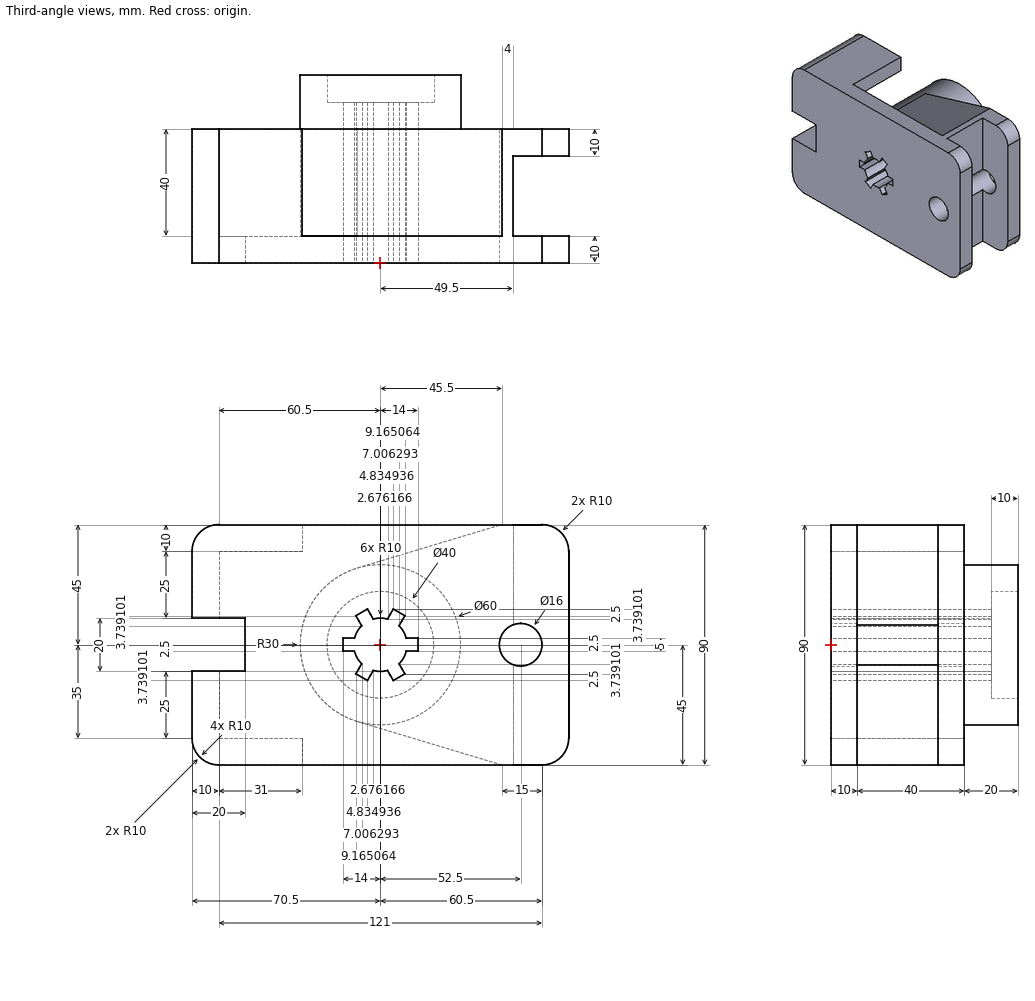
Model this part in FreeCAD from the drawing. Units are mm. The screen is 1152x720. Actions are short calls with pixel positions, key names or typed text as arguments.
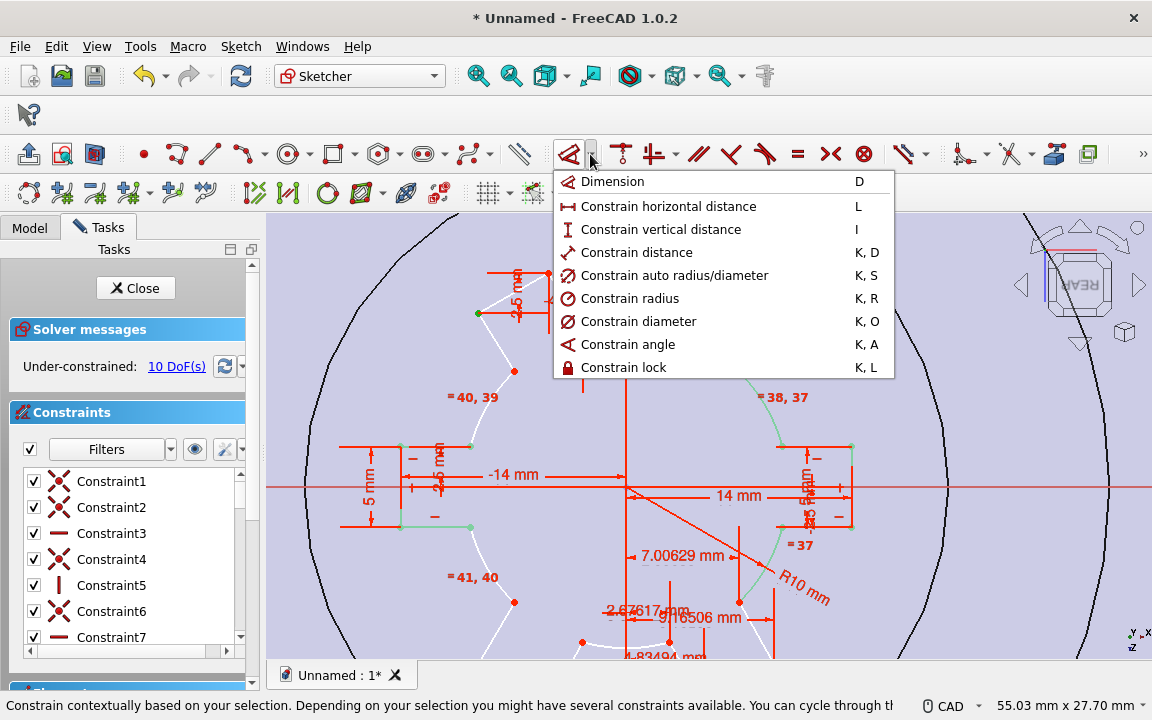
click(724, 206)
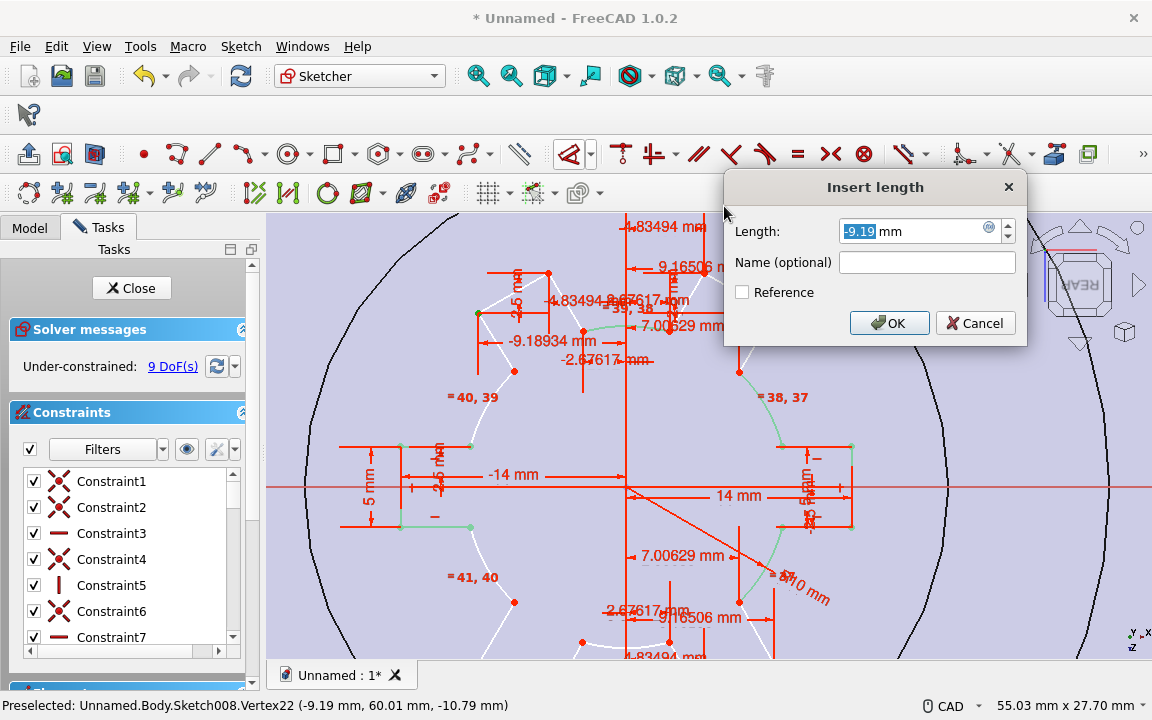
text(-9.165064)
key(Return)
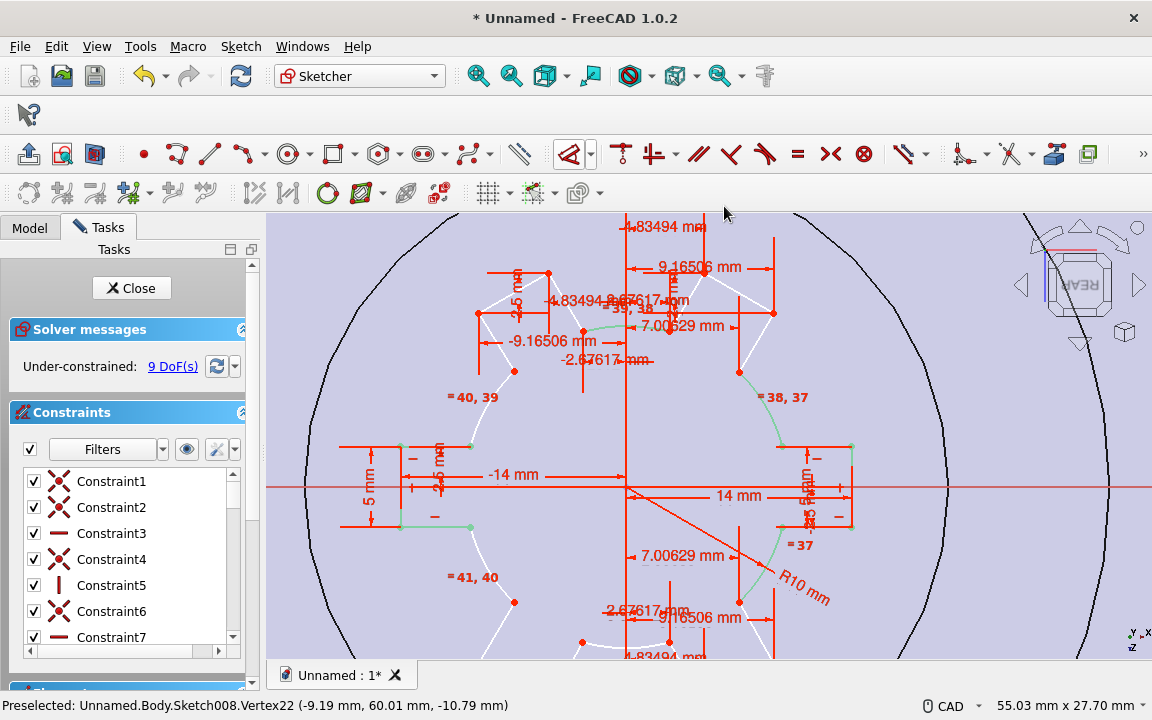
click(515, 371)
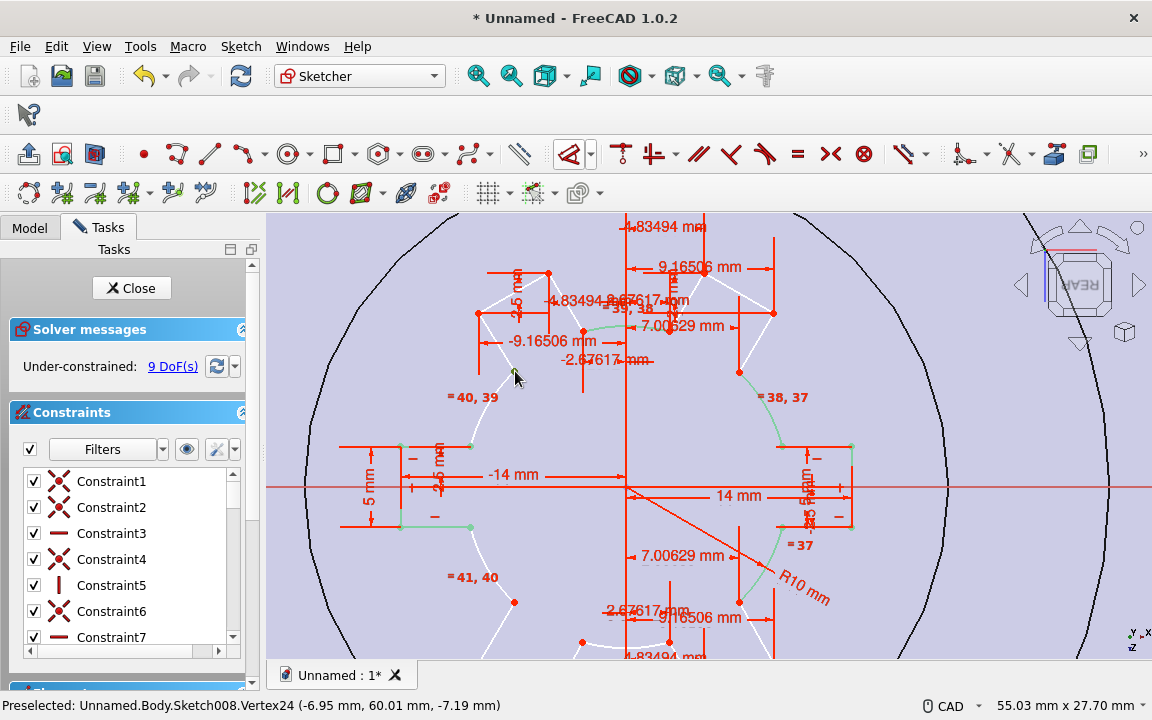
click(590, 154)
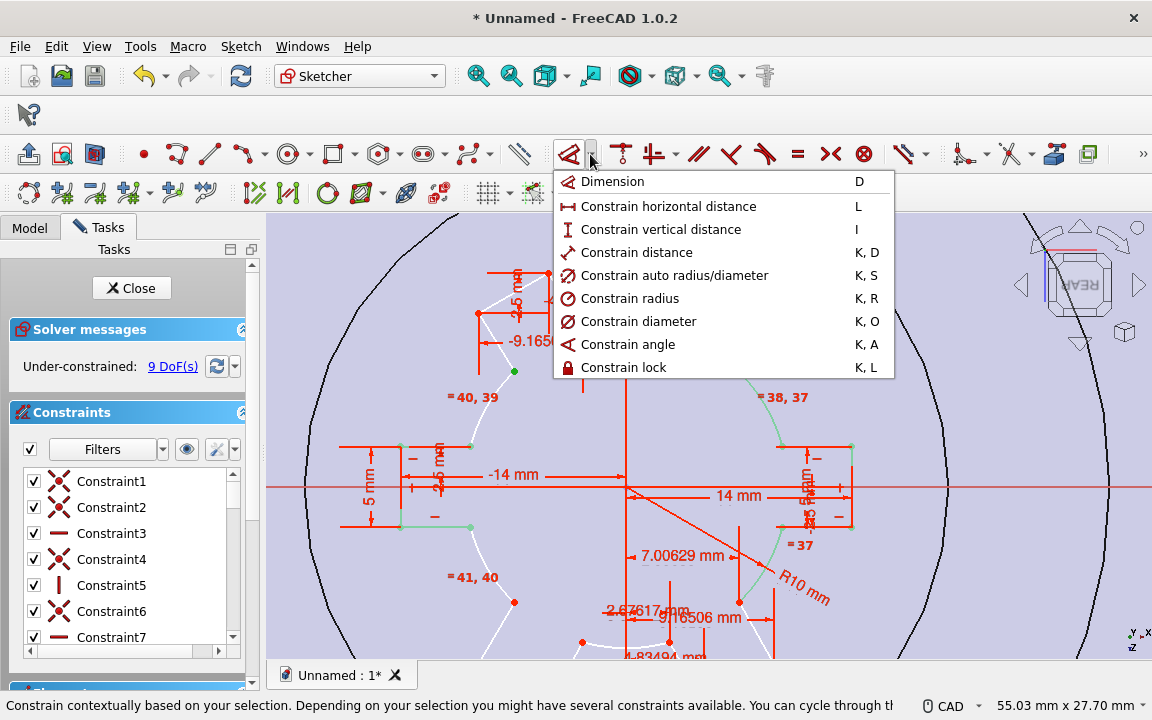
click(724, 206)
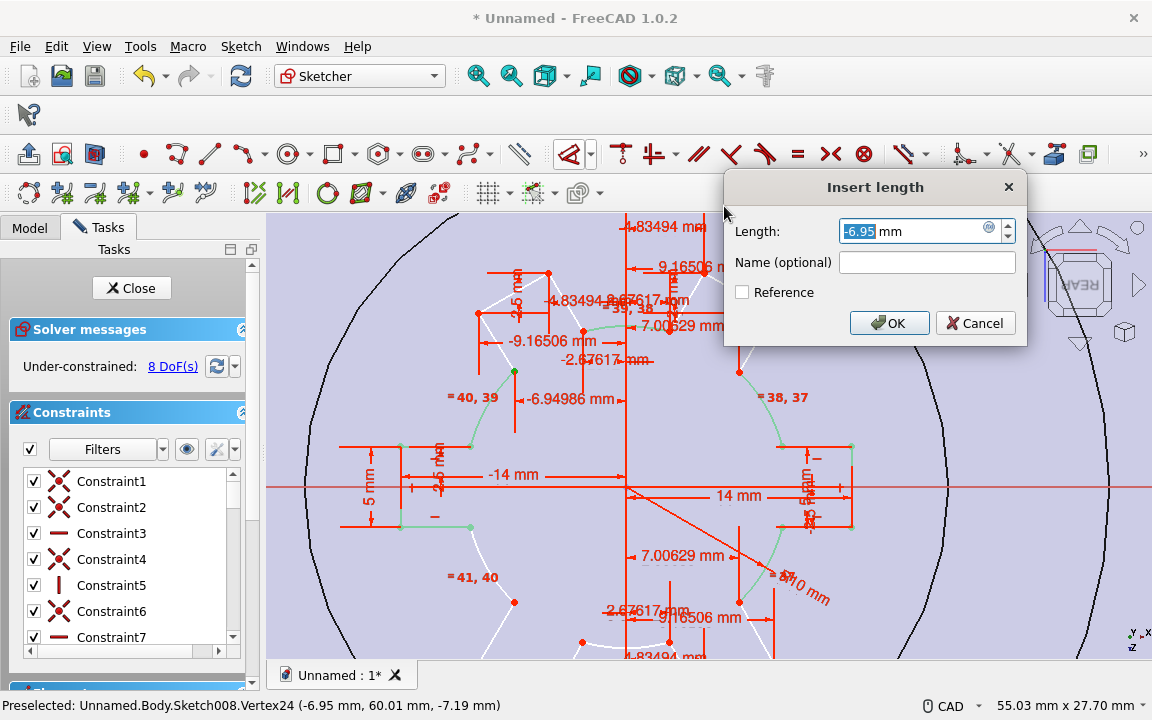
text(-7.006293)
key(Return)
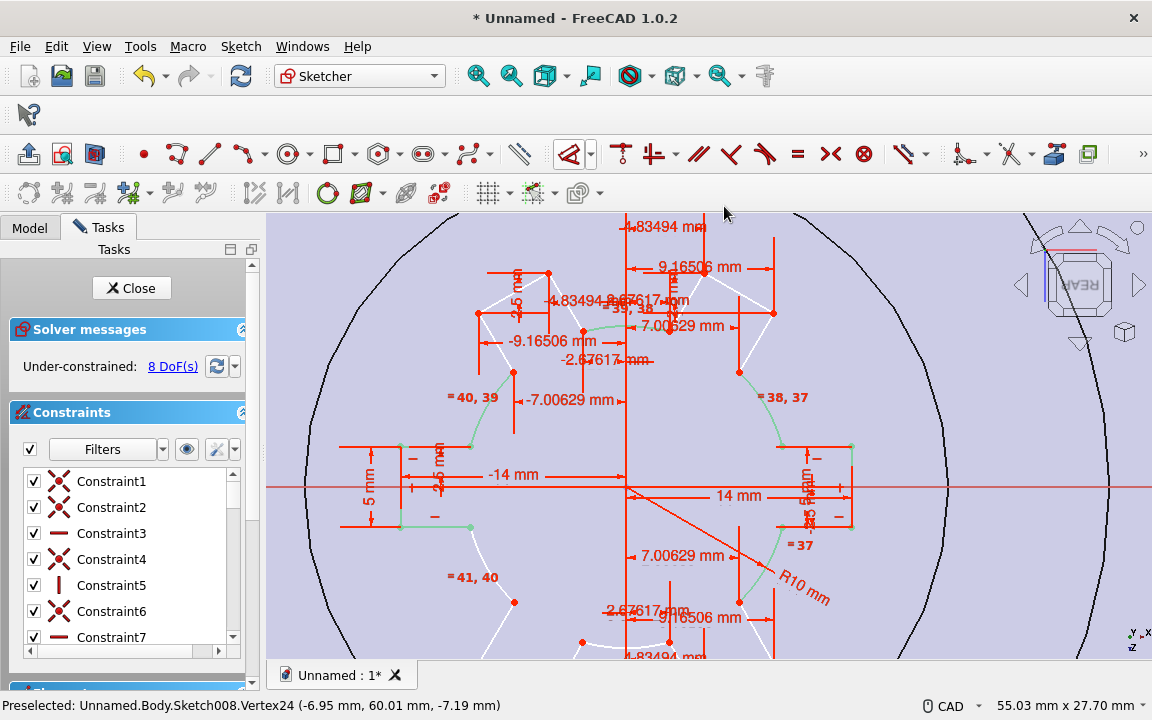
click(514, 603)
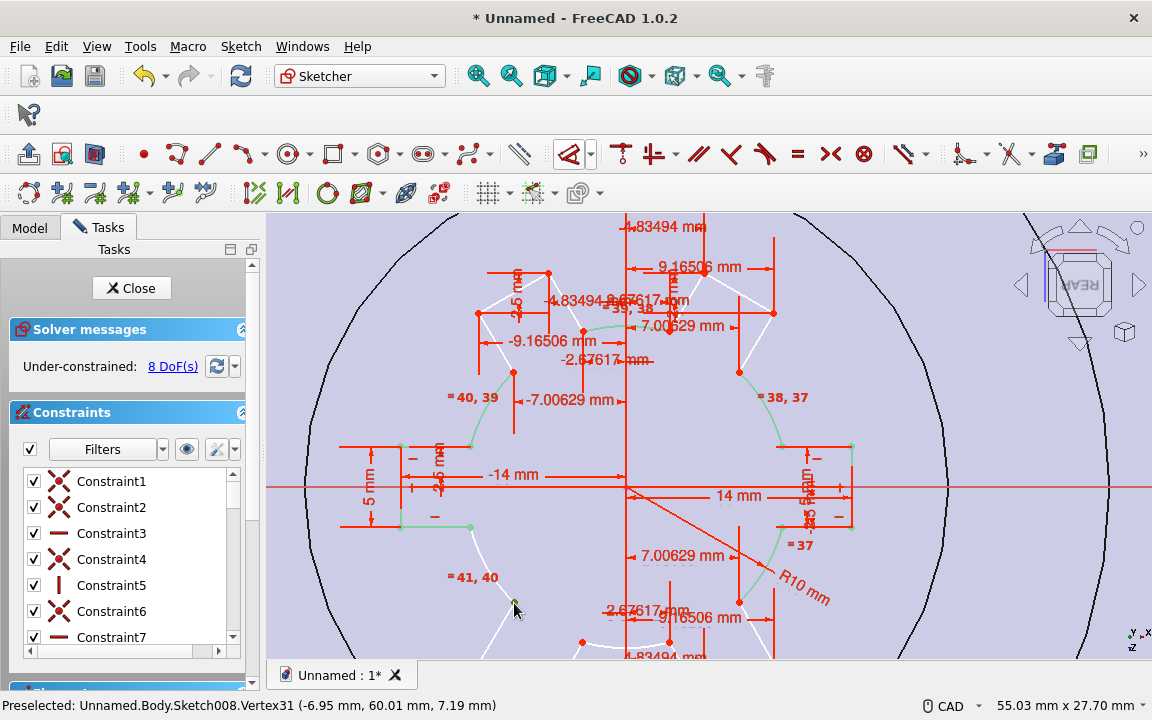
click(590, 154)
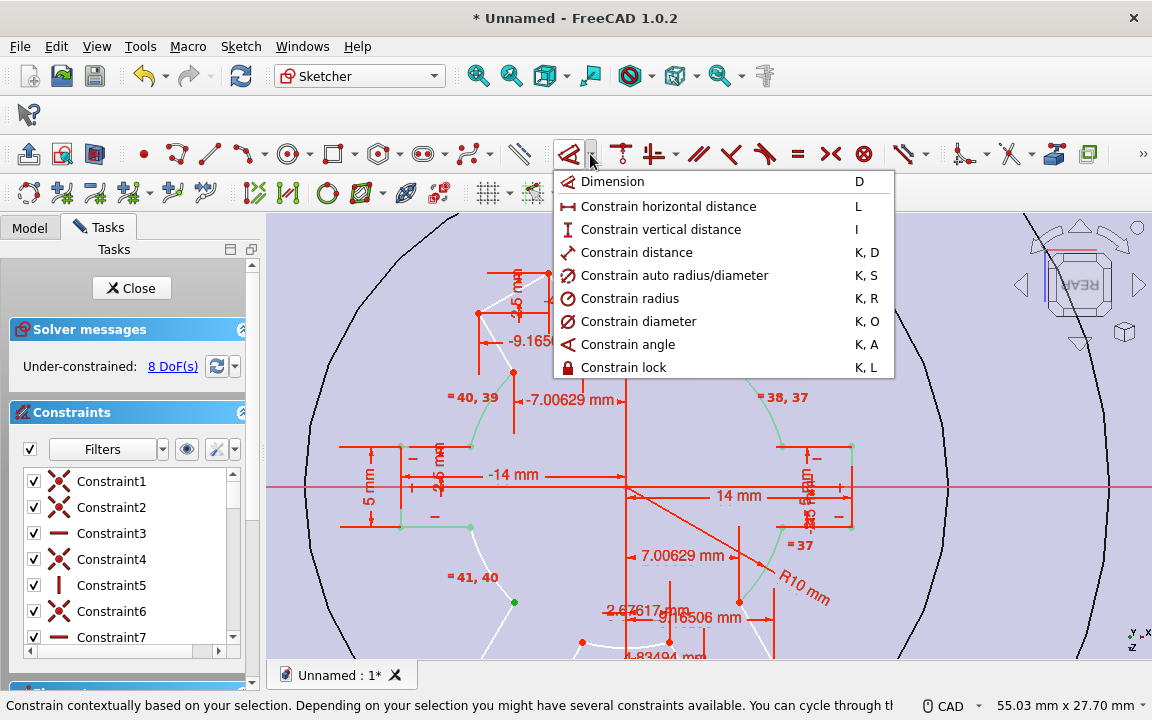
click(724, 206)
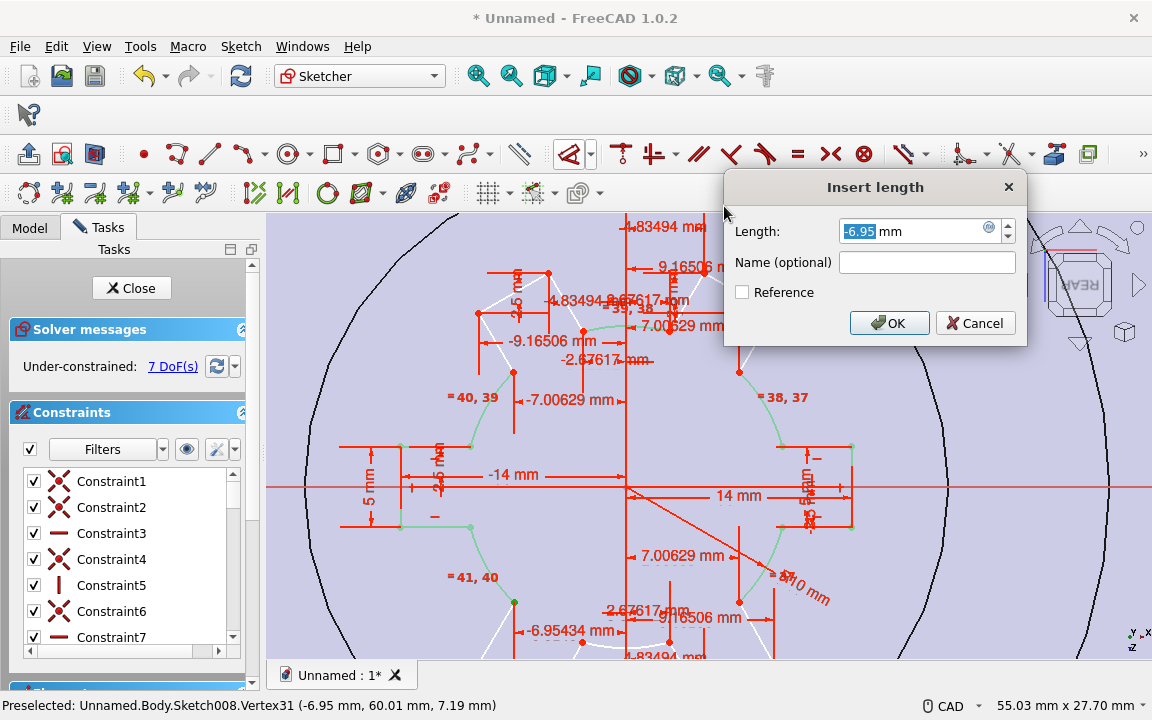
text(-7.006293)
key(Return)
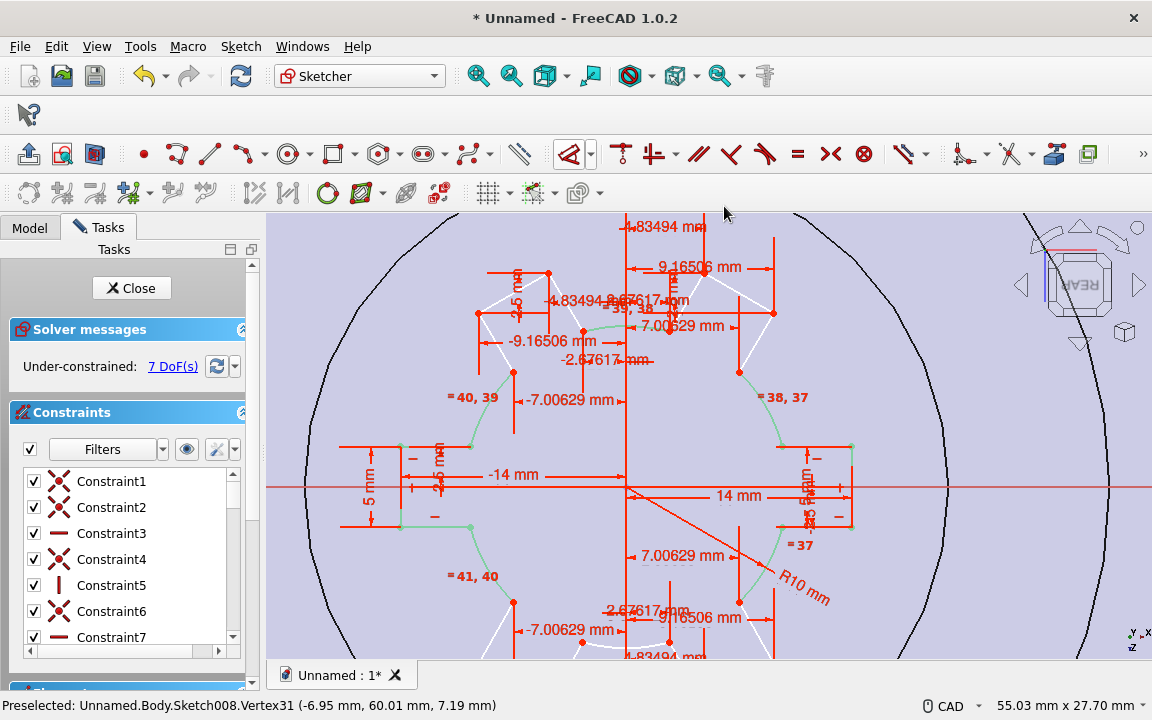
scroll(669, 332, down, 2)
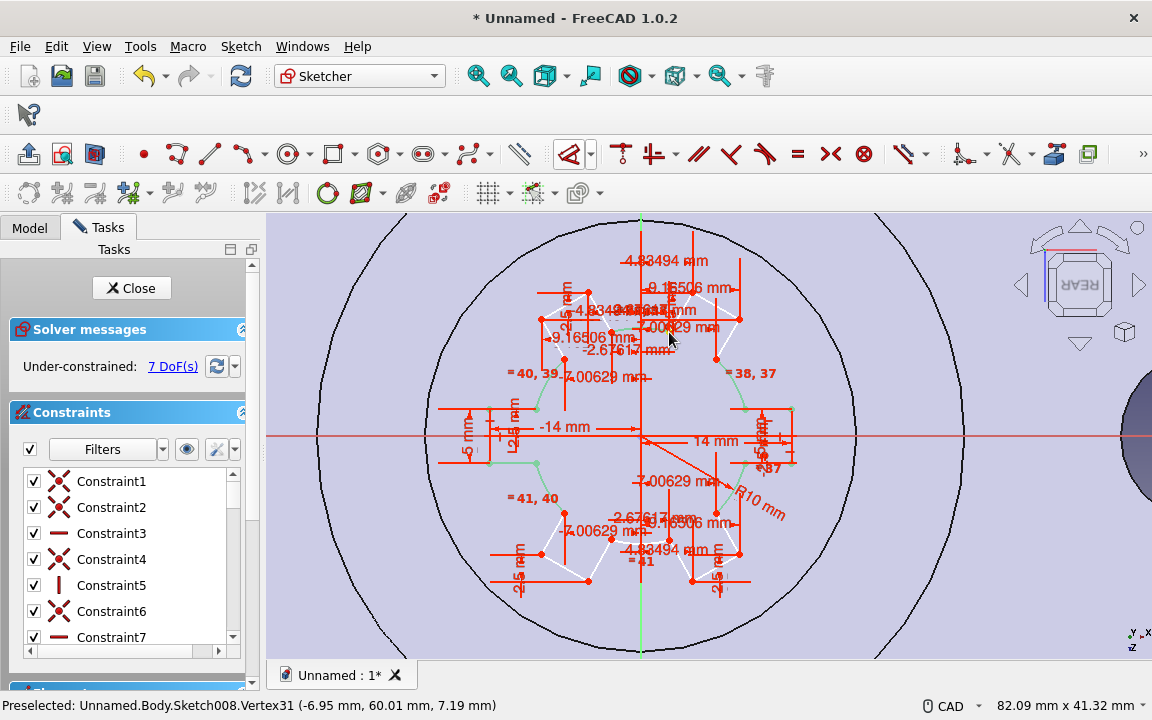
click(541, 555)